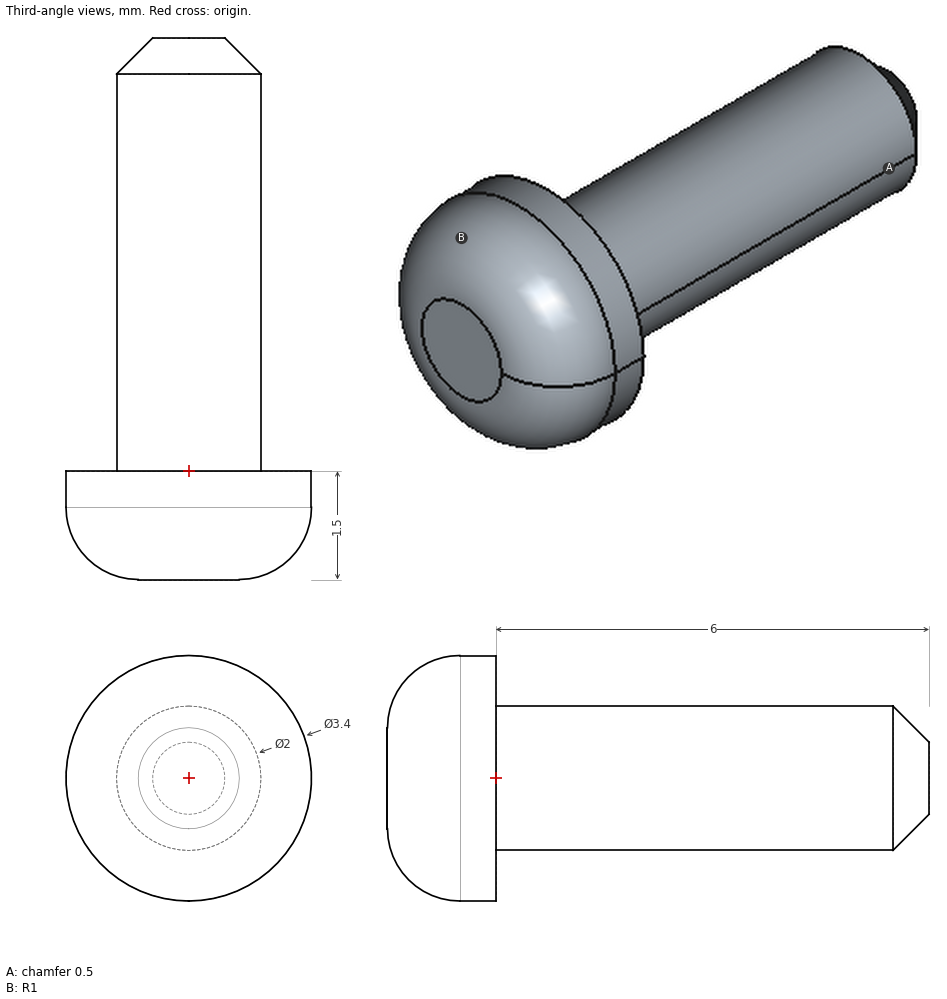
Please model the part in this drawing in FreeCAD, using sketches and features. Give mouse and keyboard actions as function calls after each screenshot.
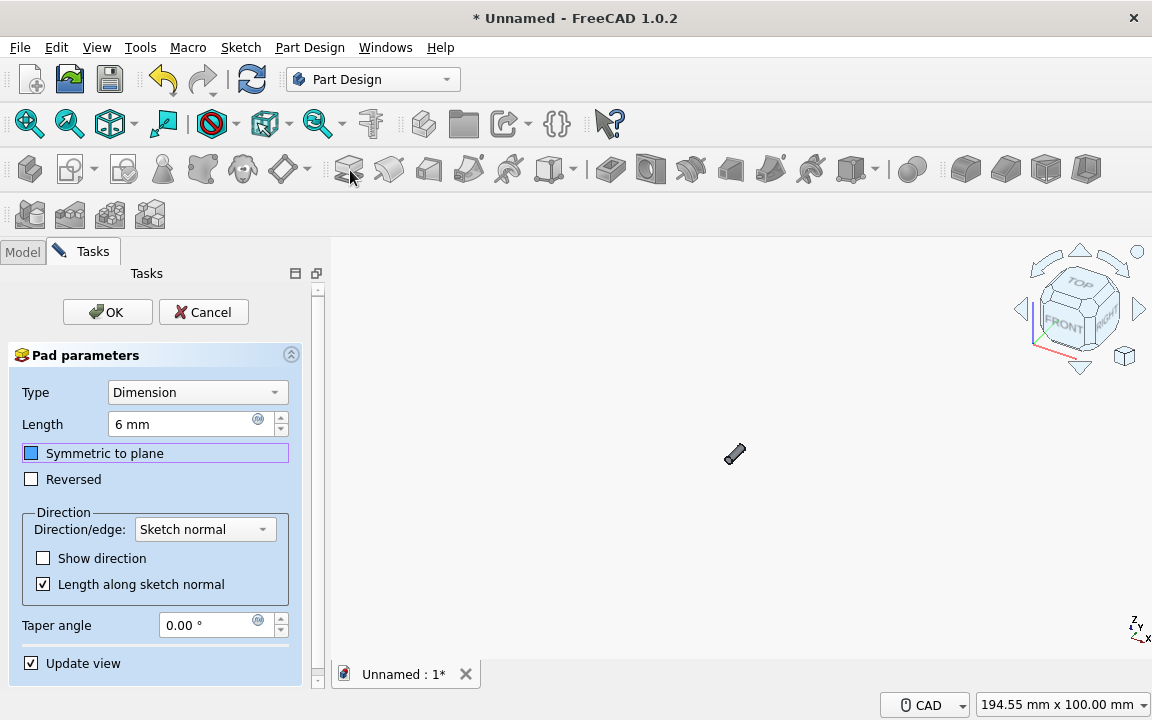
click(30, 479)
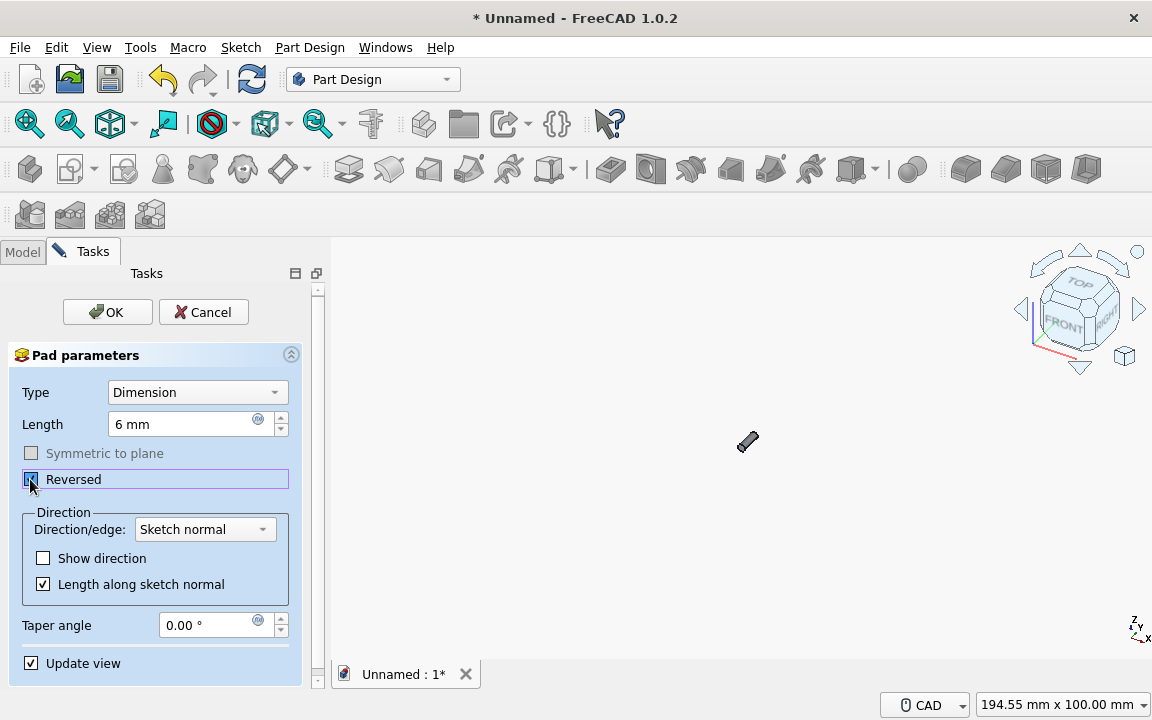
click(108, 312)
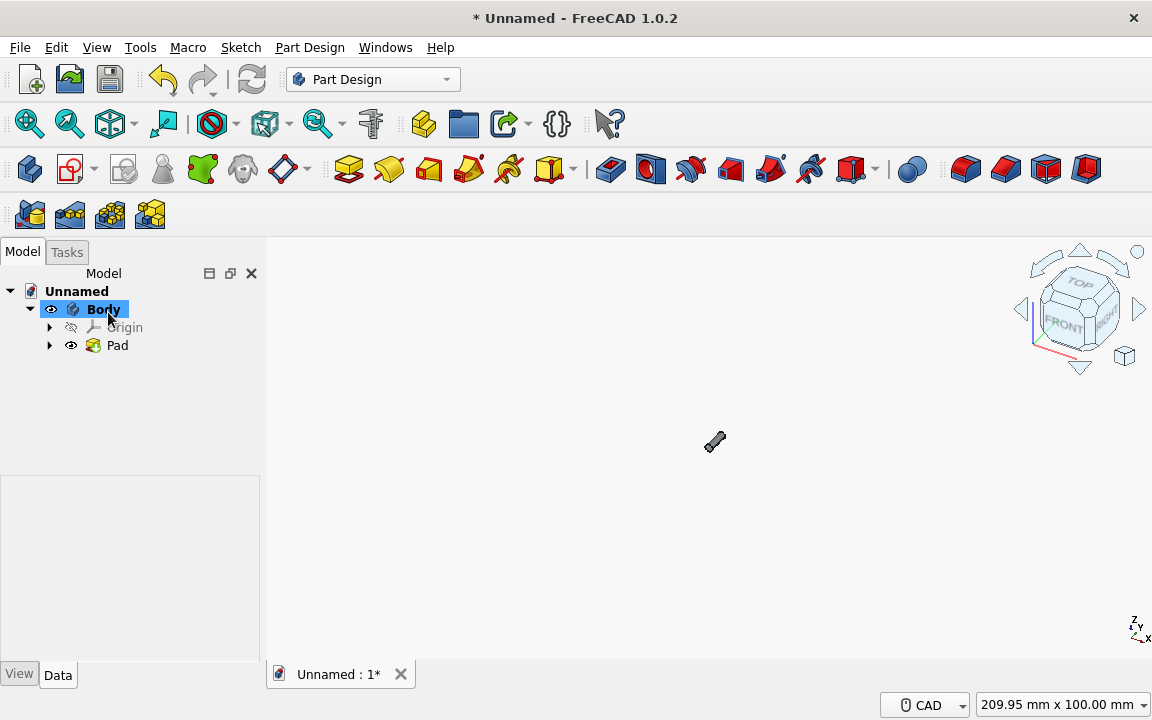
click(30, 124)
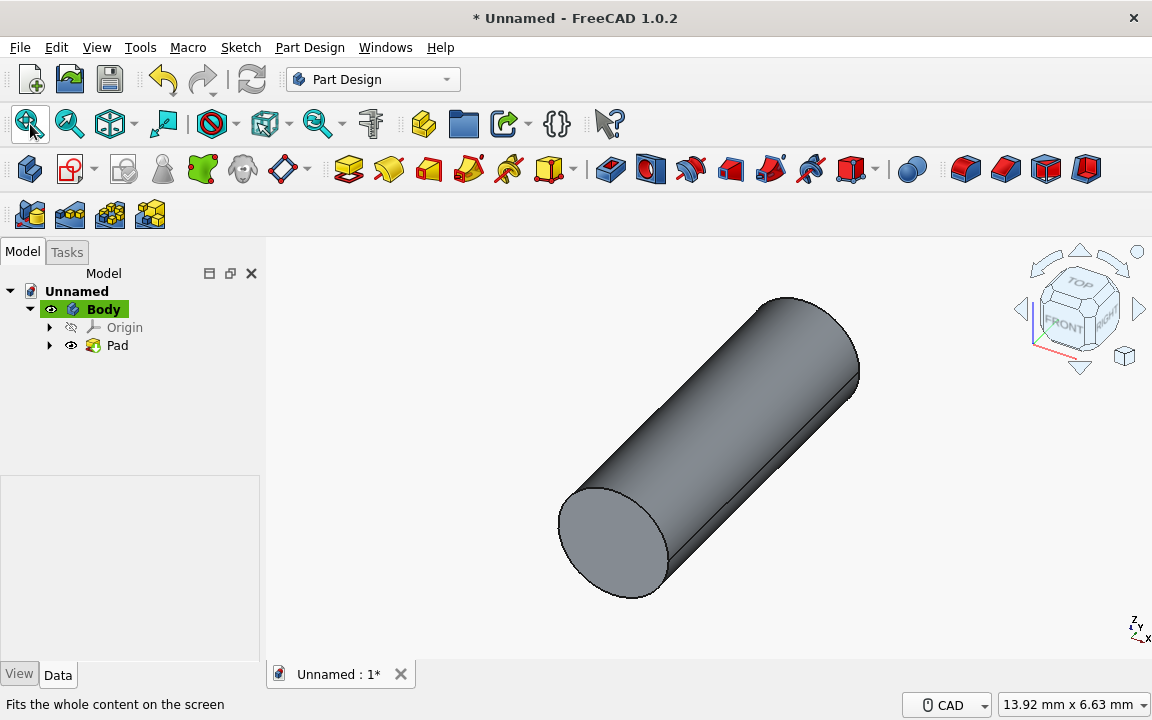
key(0)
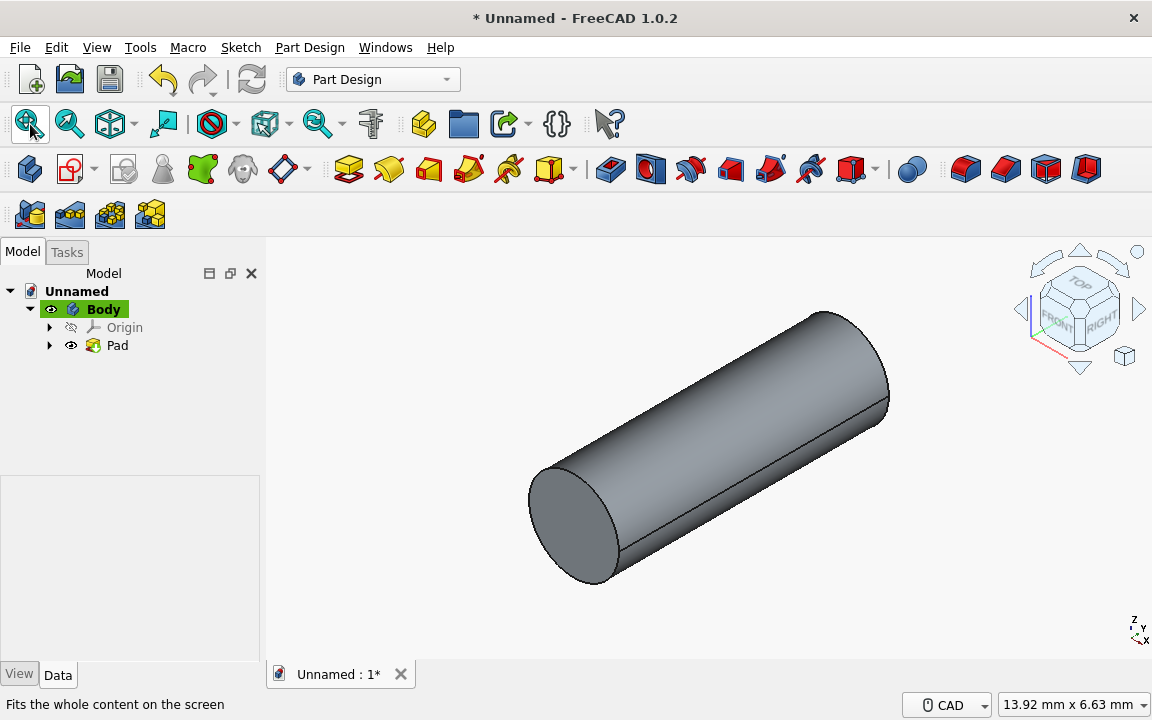
key(2)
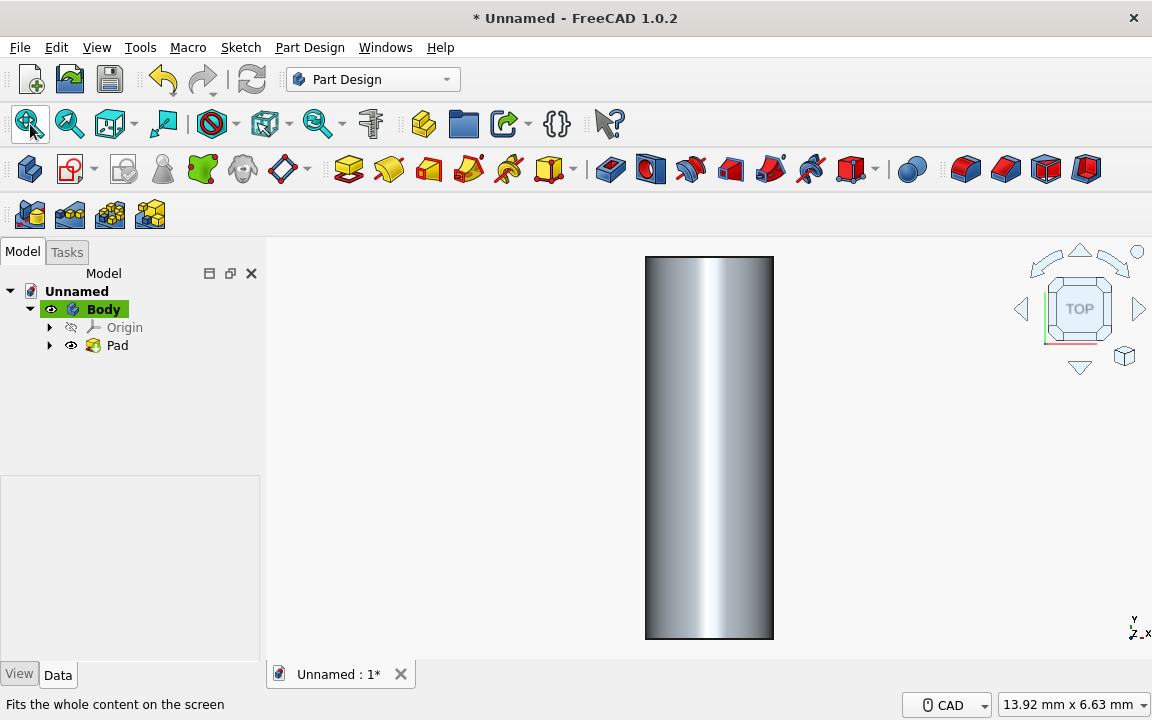
key(1)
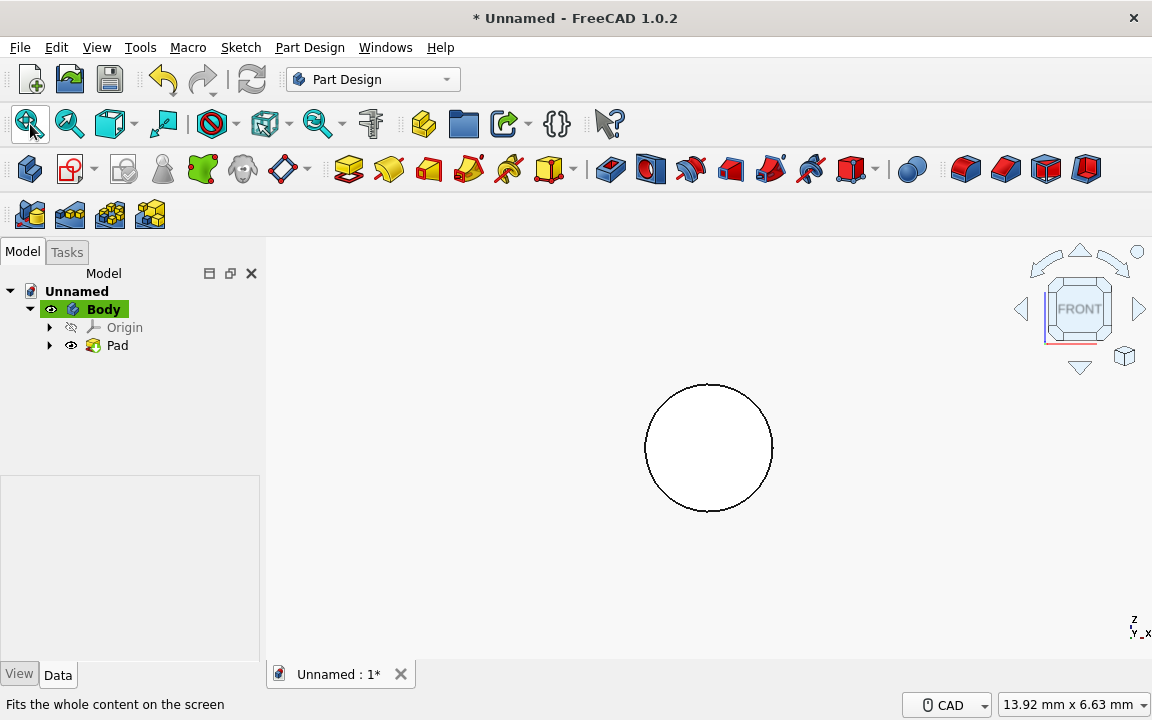
click(30, 124)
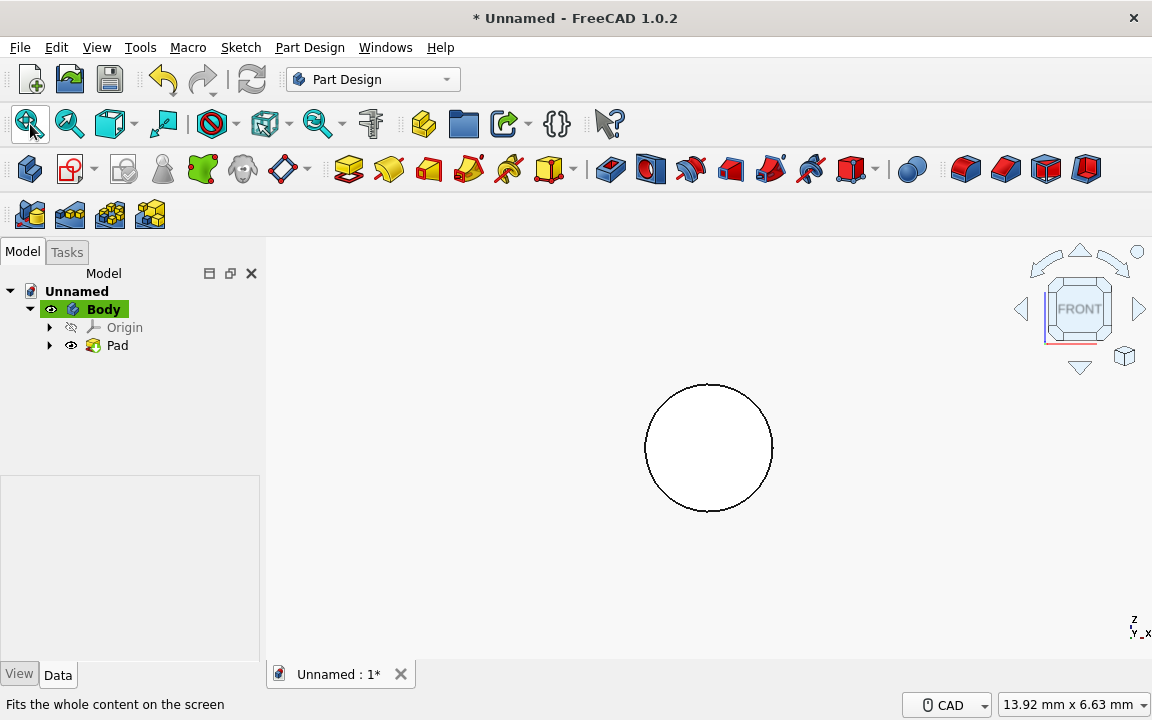
key(3)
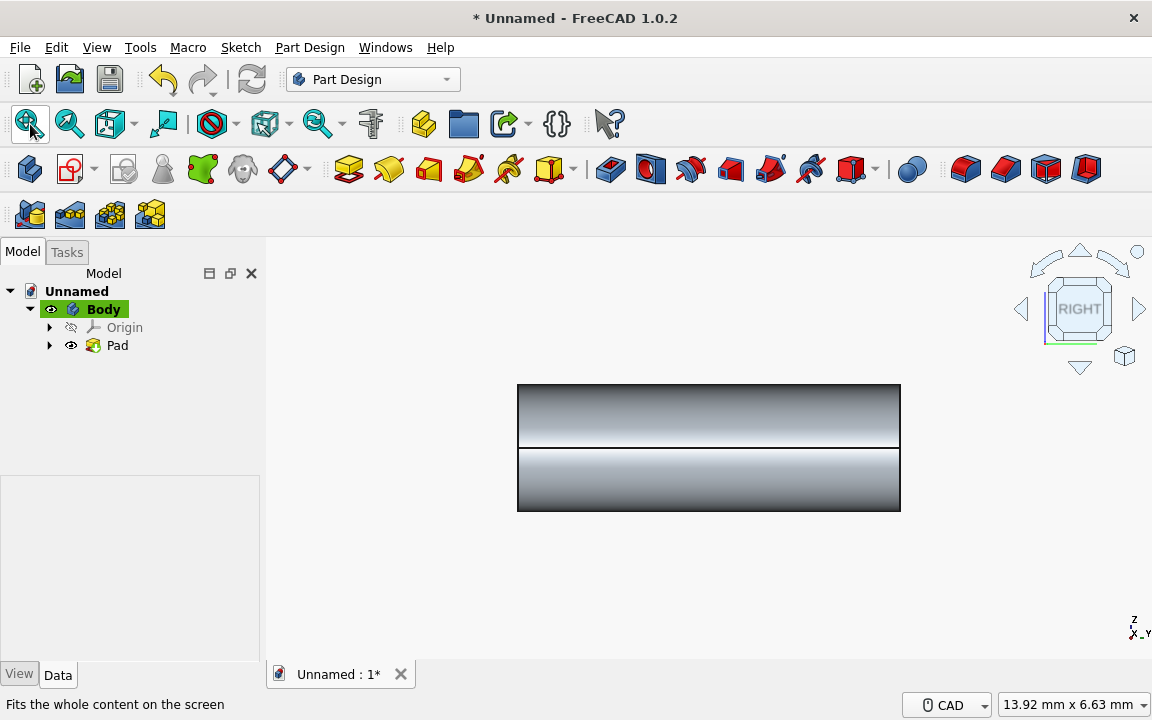
click(30, 124)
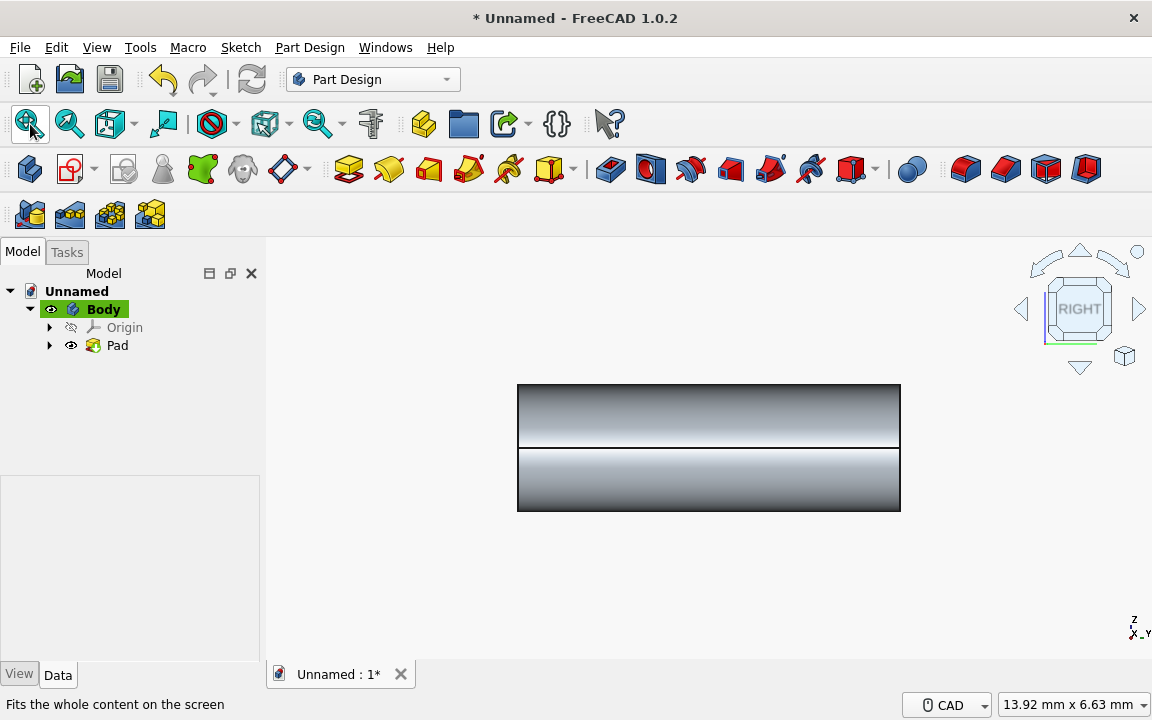
click(900, 410)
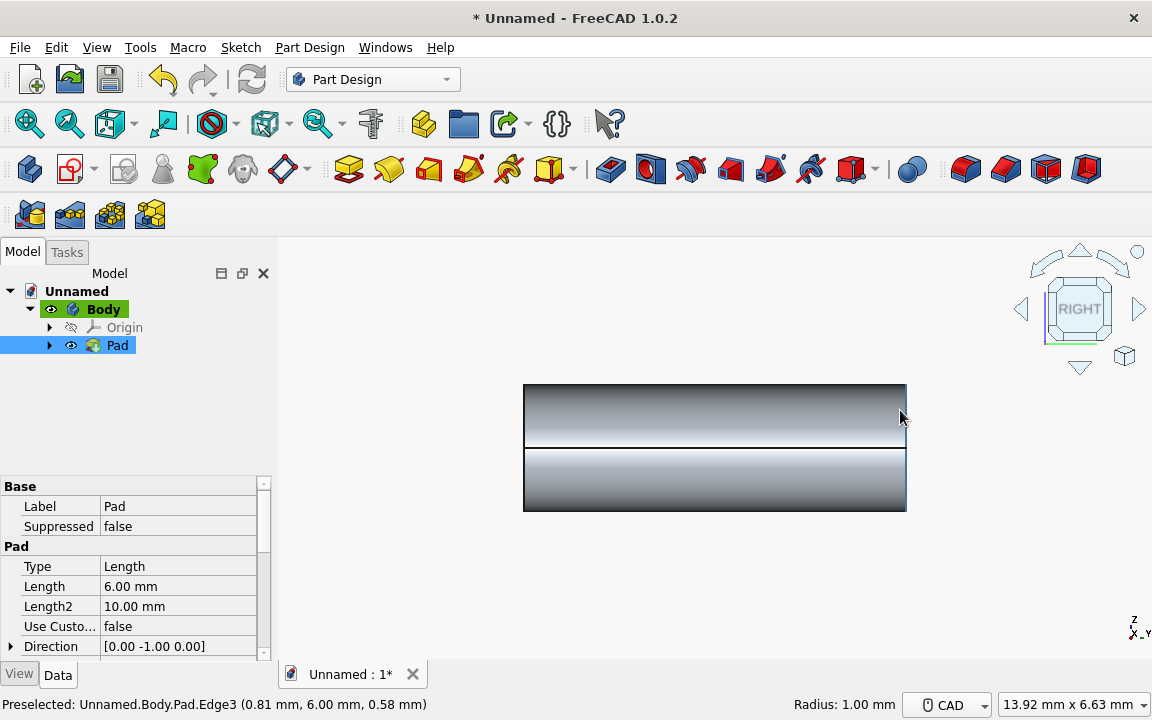
click(1006, 170)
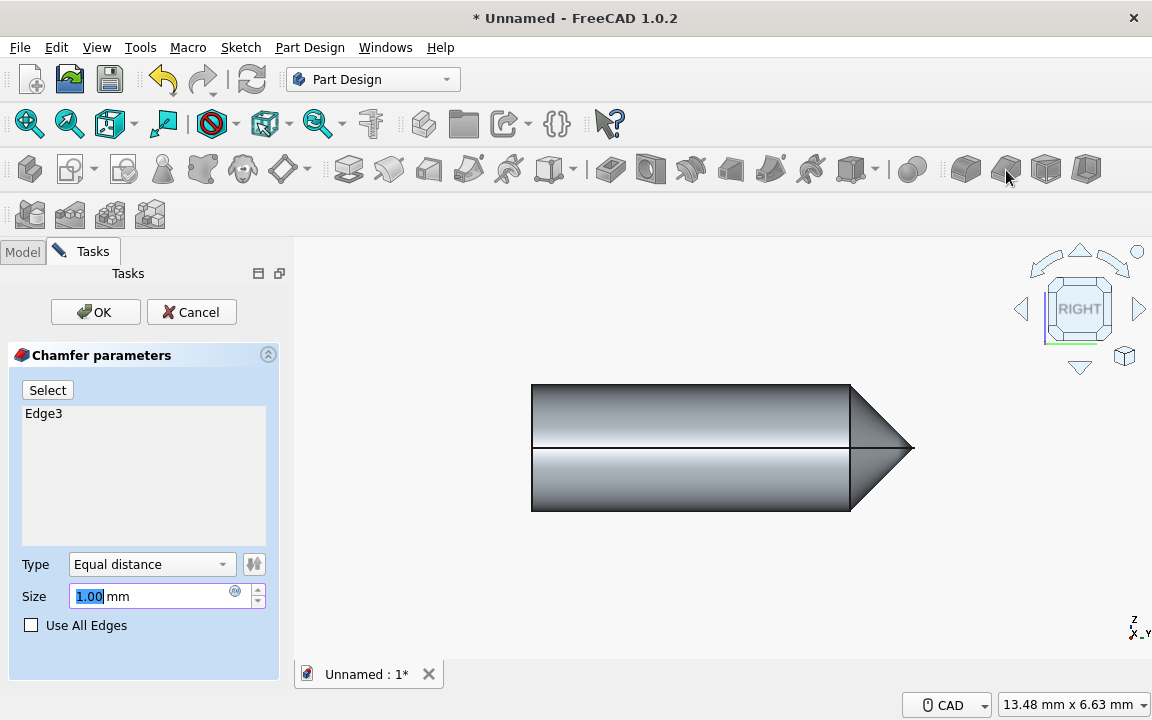
text(0.5)
key(Tab)